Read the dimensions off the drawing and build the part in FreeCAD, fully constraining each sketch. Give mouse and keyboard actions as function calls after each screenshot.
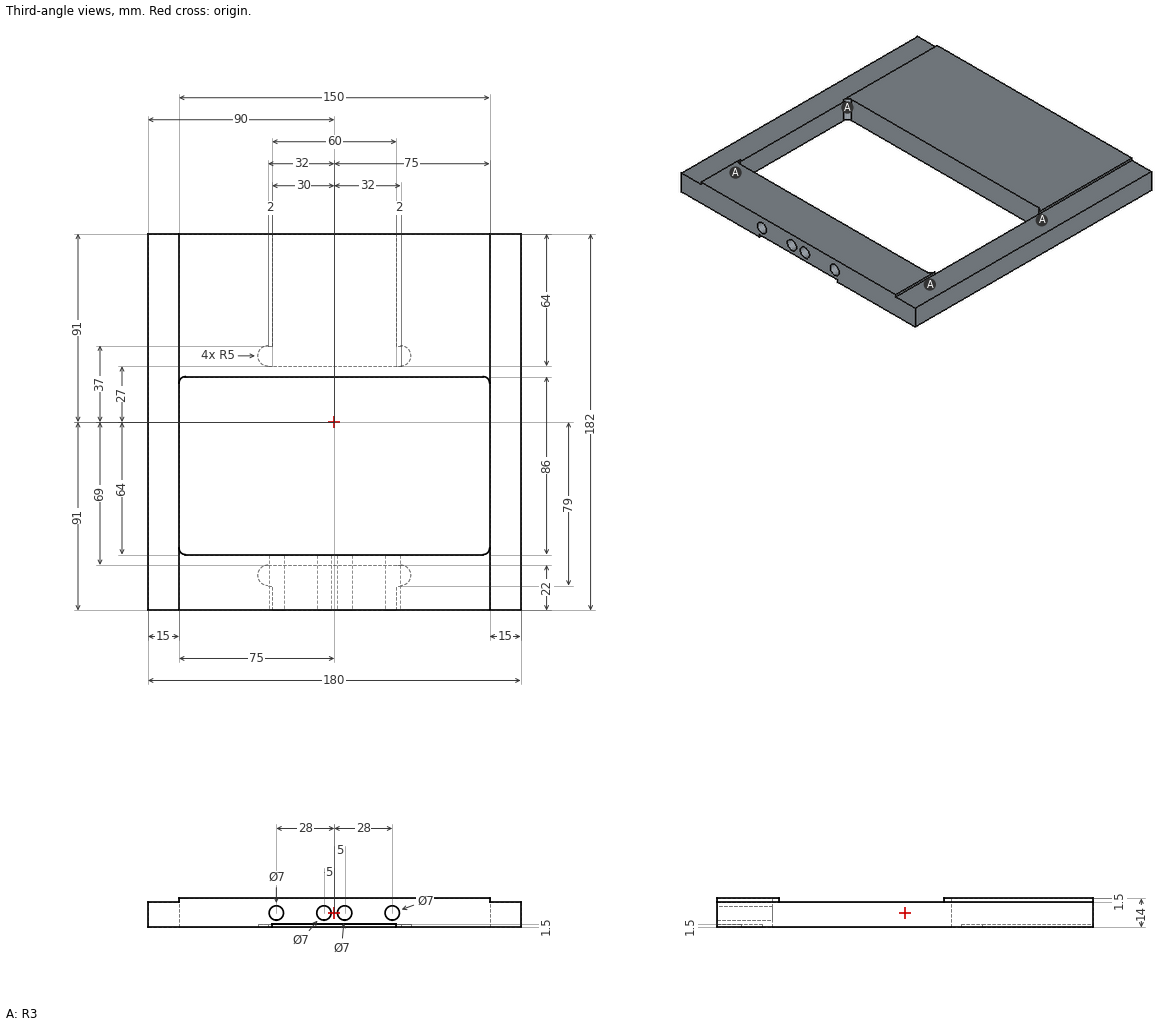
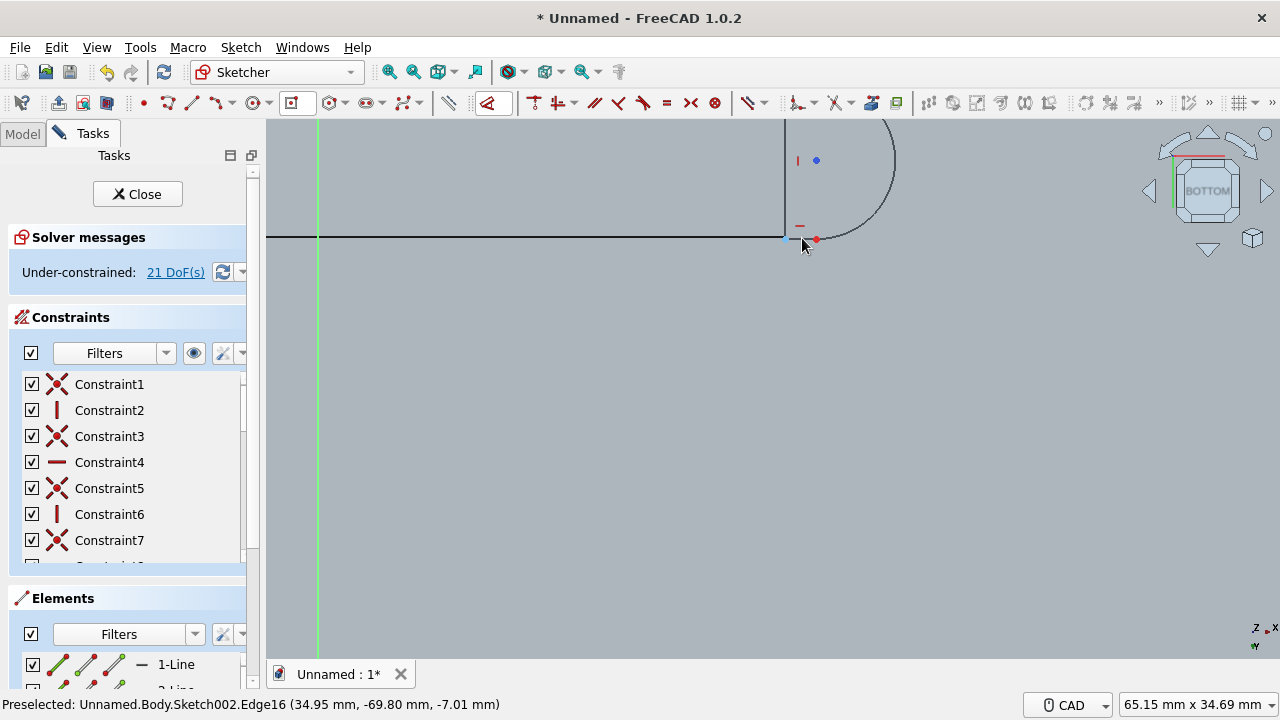
click(801, 239)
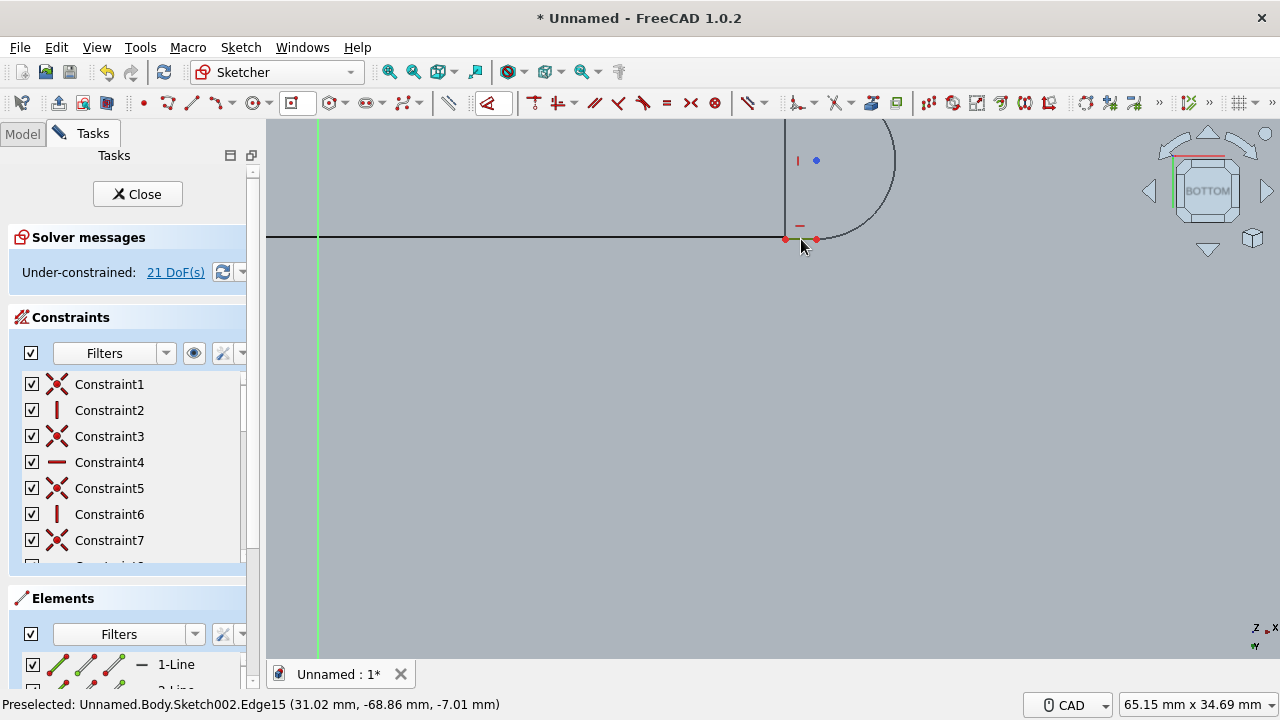
scroll(802, 239, down, 8)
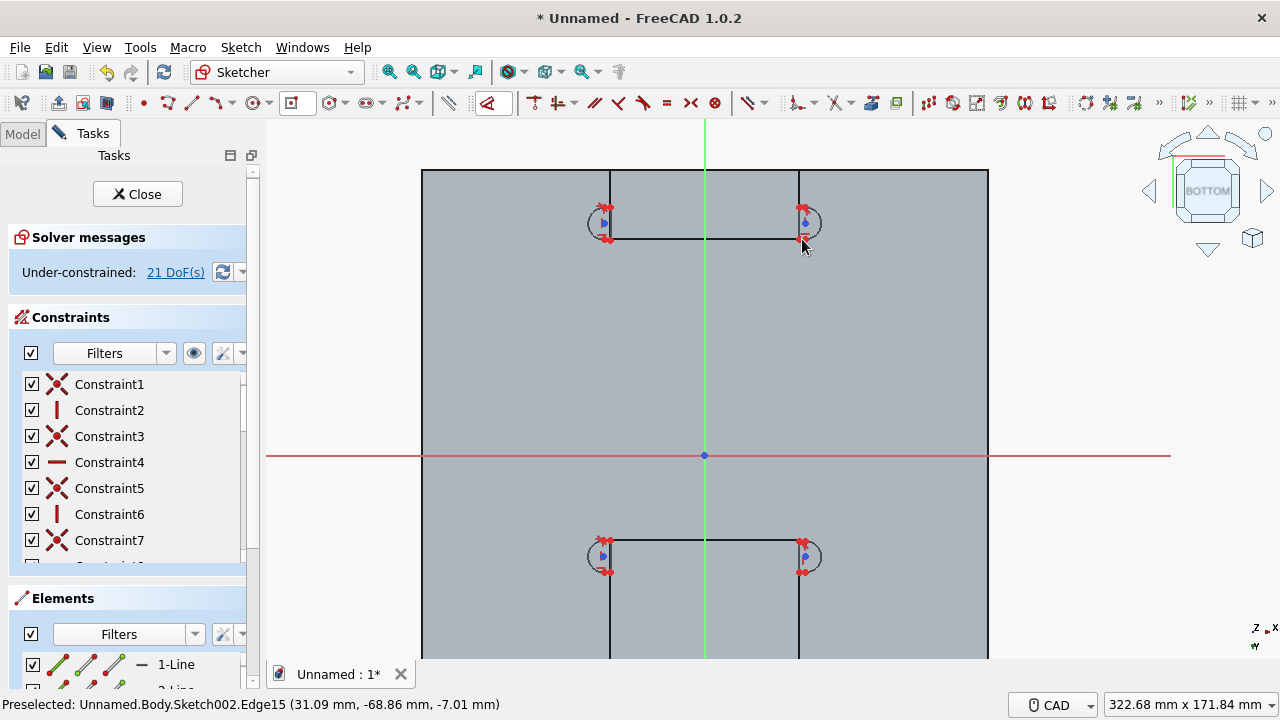
click(818, 233)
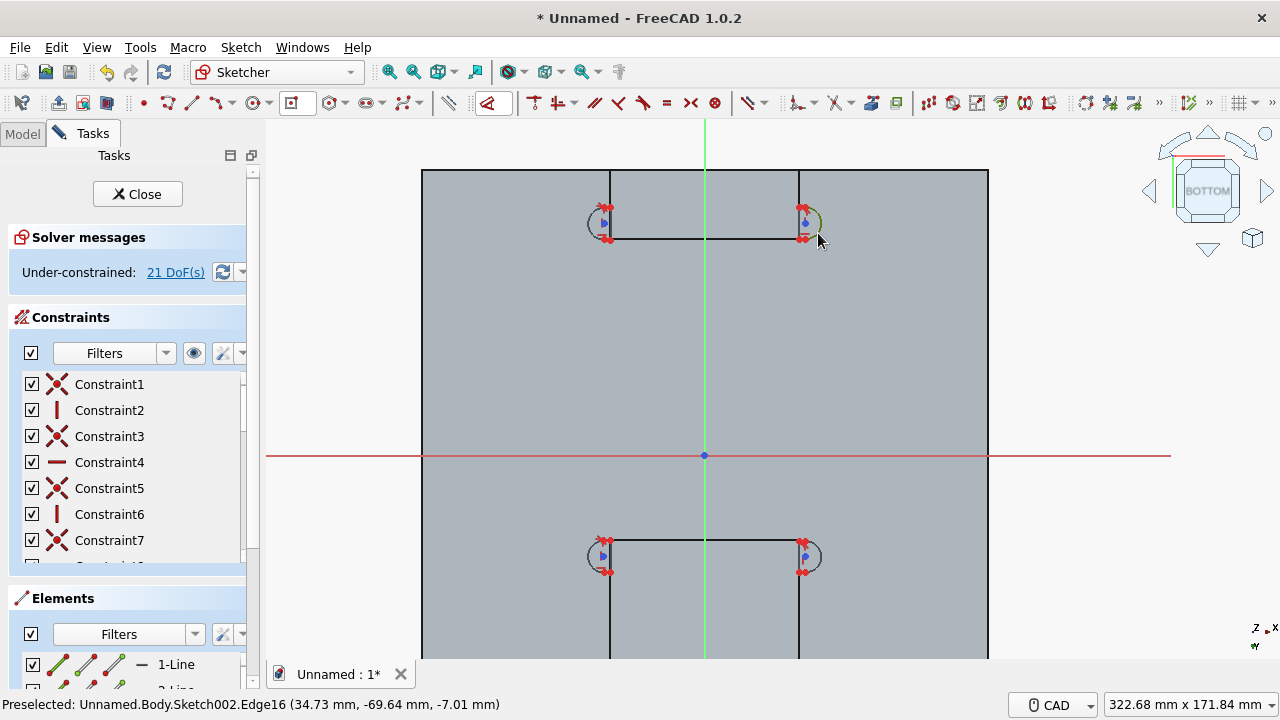
click(644, 104)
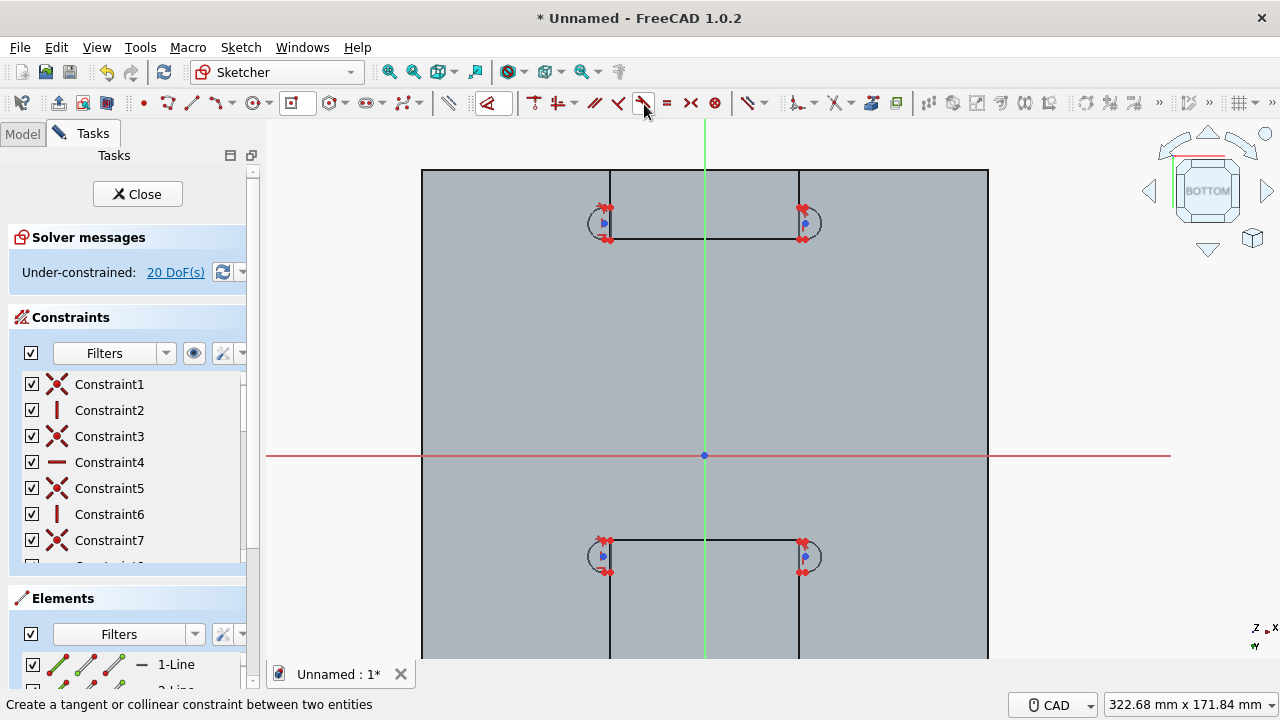
scroll(608, 572, up, 8)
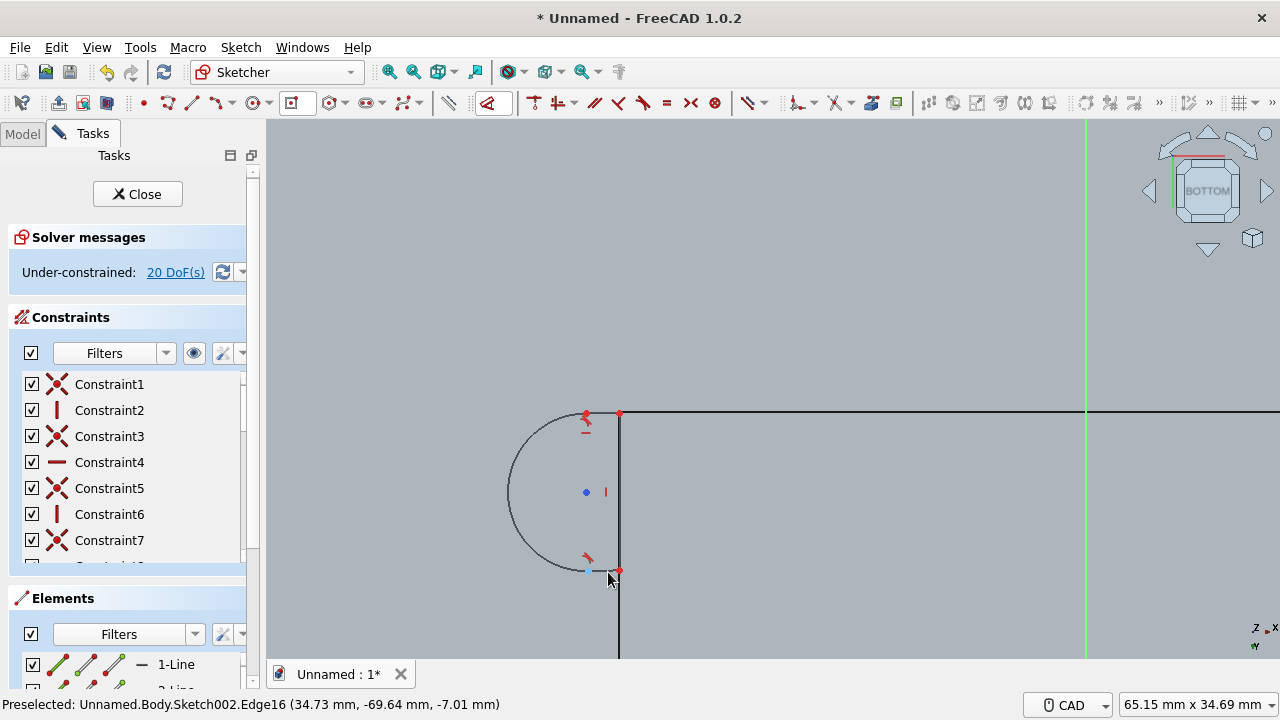
click(604, 571)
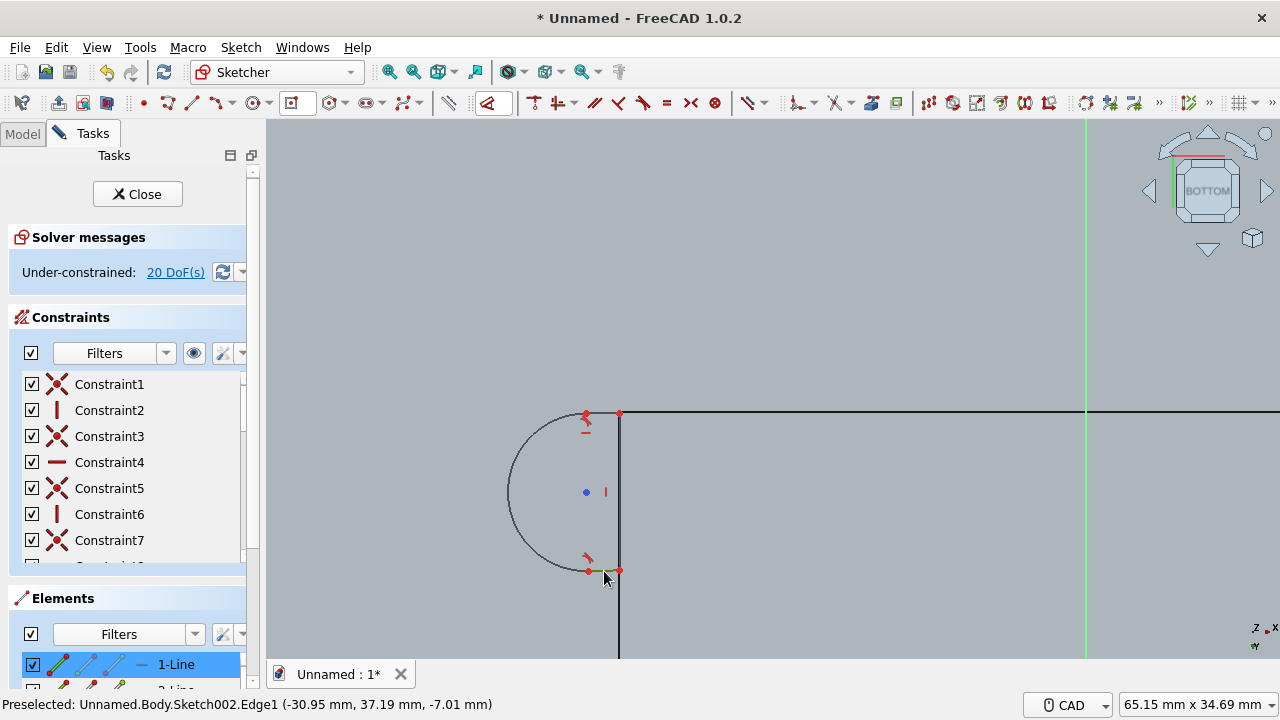
key(h)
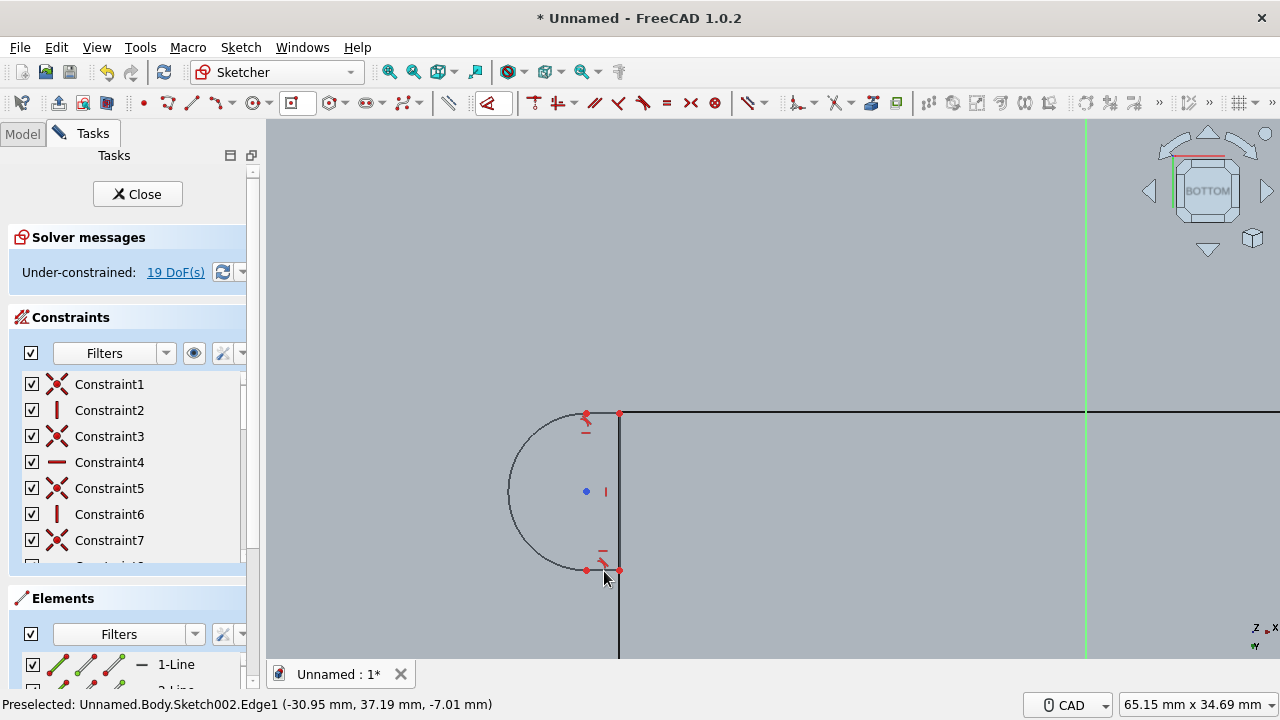
scroll(608, 572, down, 8)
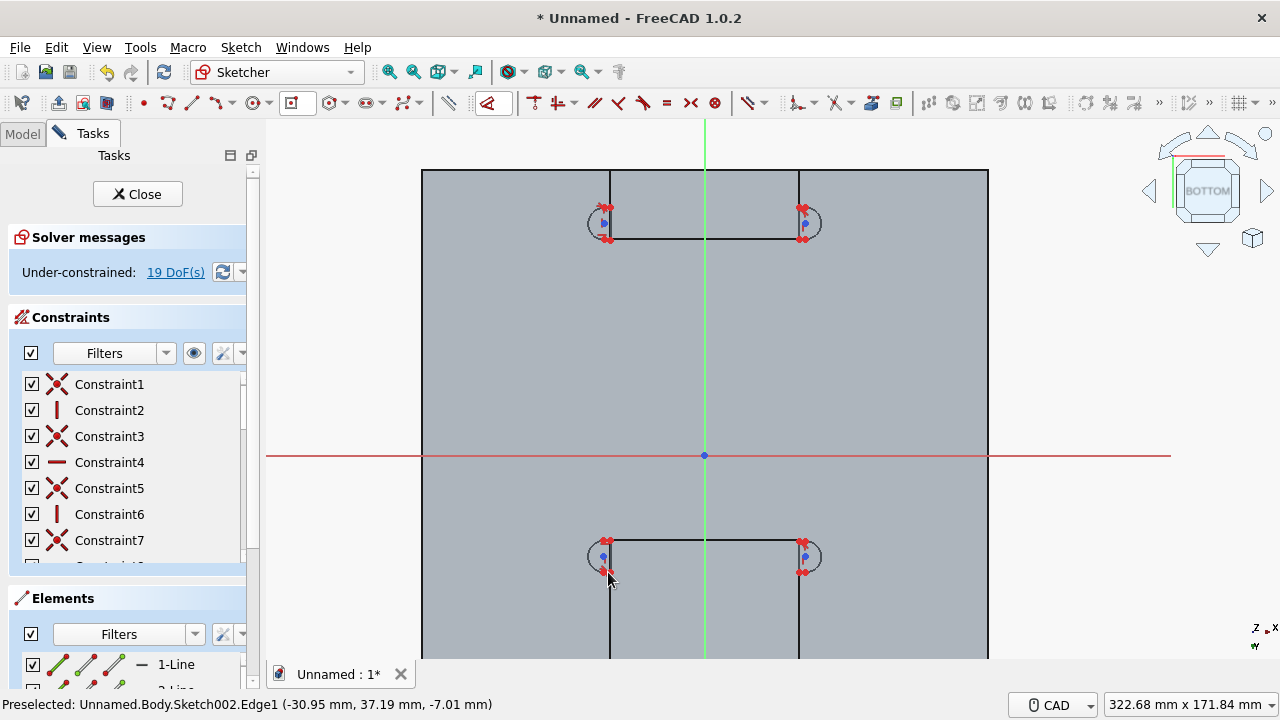
scroll(803, 541, up, 11)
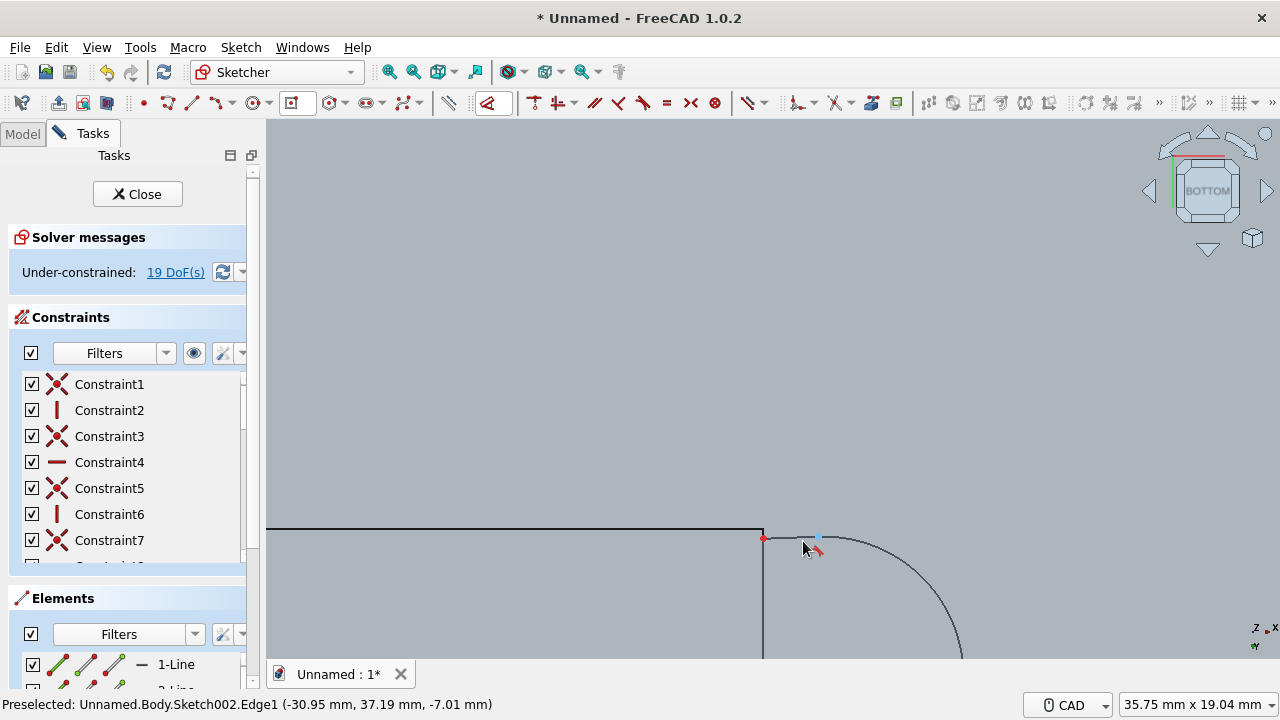
click(802, 537)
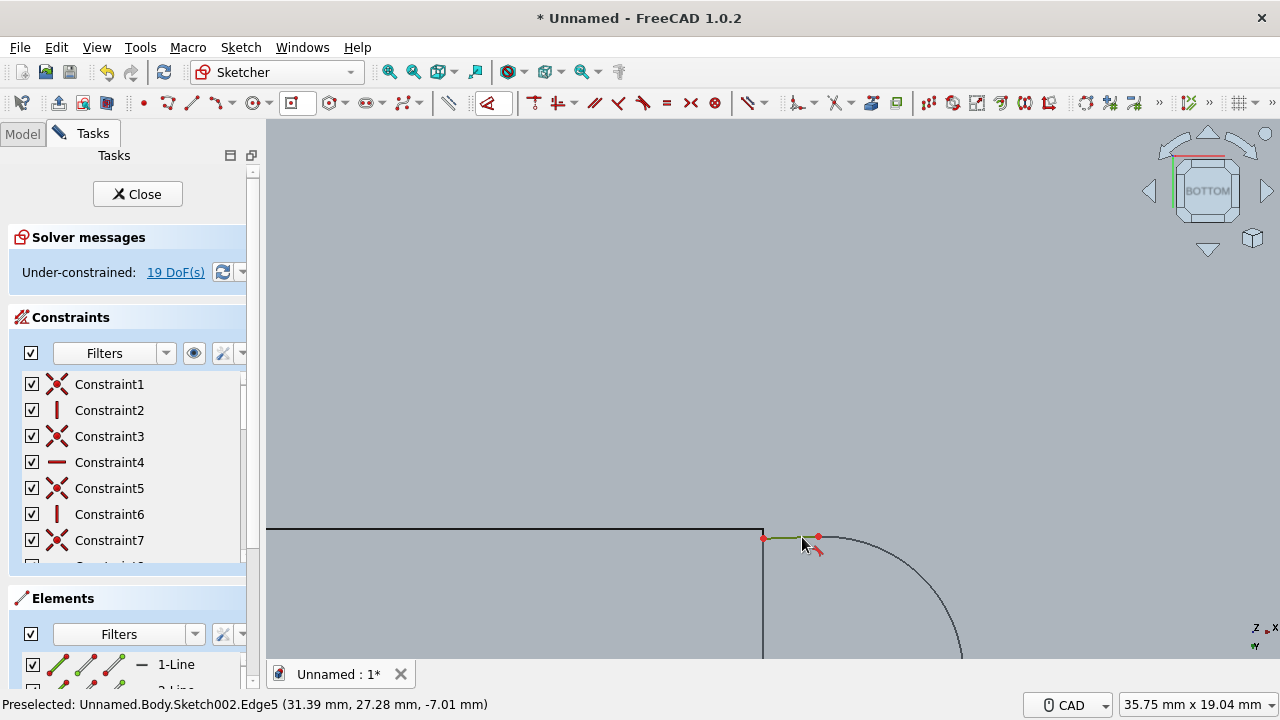
key(h)